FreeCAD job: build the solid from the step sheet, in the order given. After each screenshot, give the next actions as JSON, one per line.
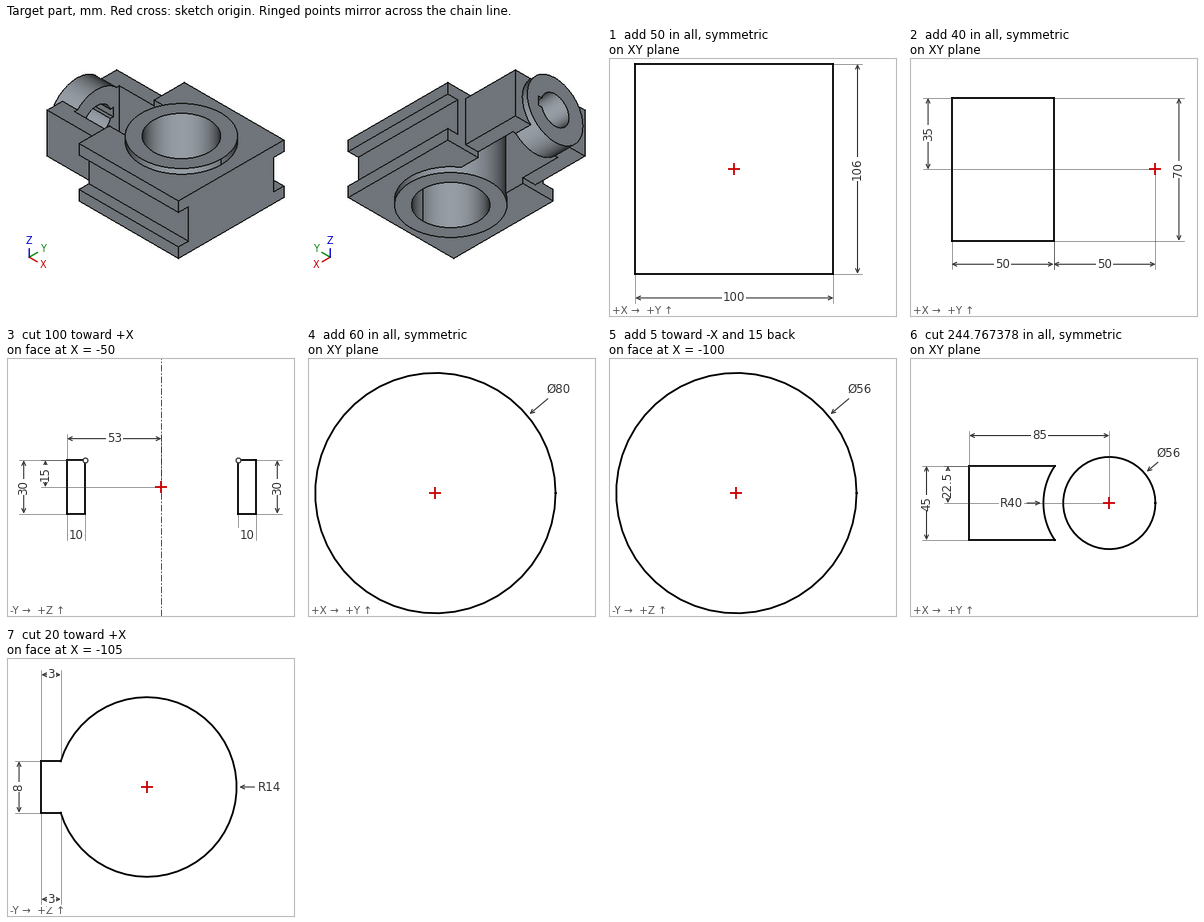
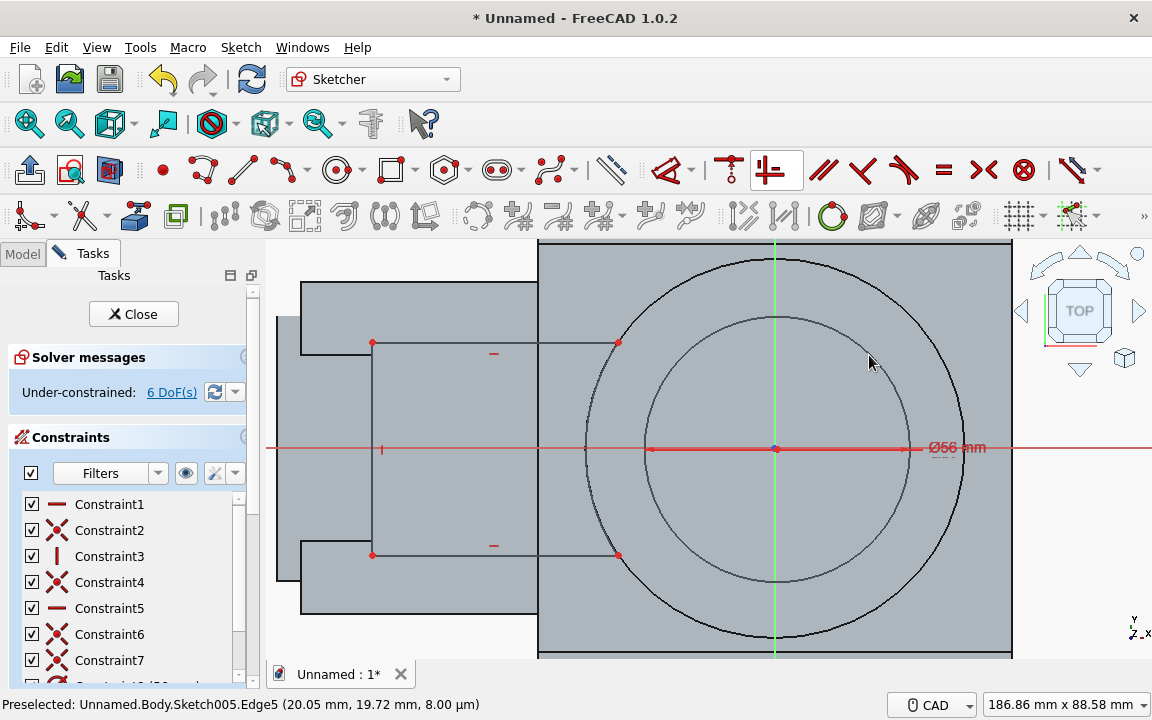
{"action": "left_click_drag", "start_coordinate": [765, 438], "coordinate": [787, 460]}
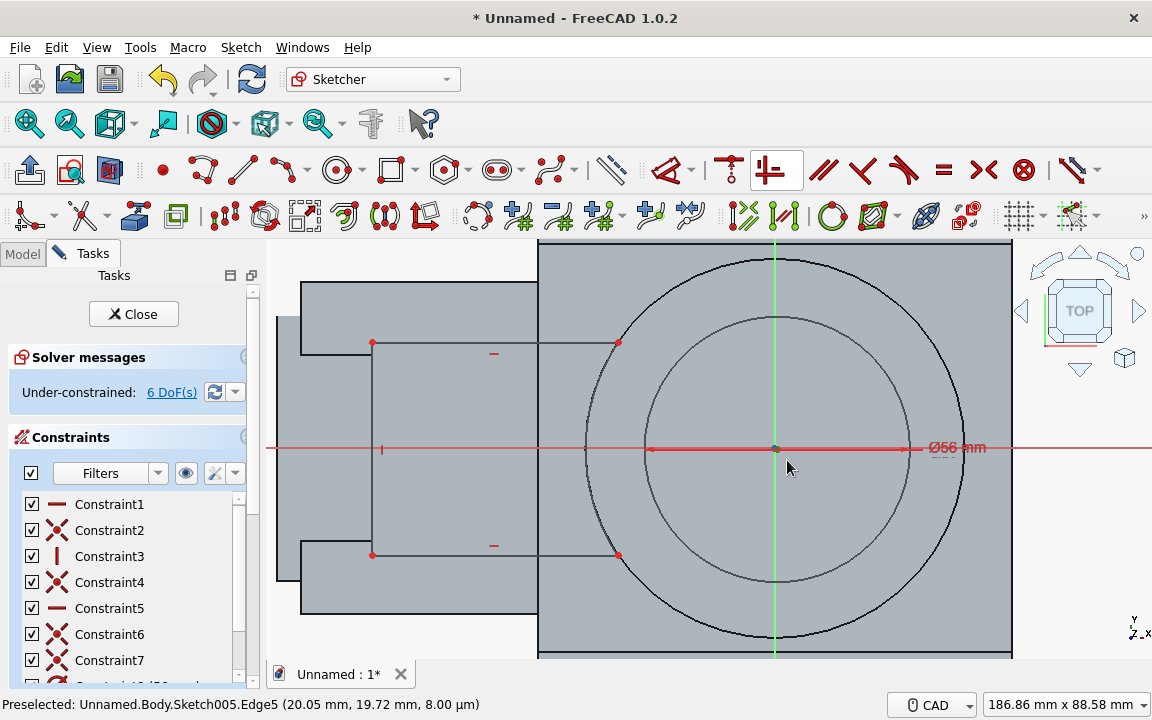
{"action": "left_click", "coordinate": [730, 170]}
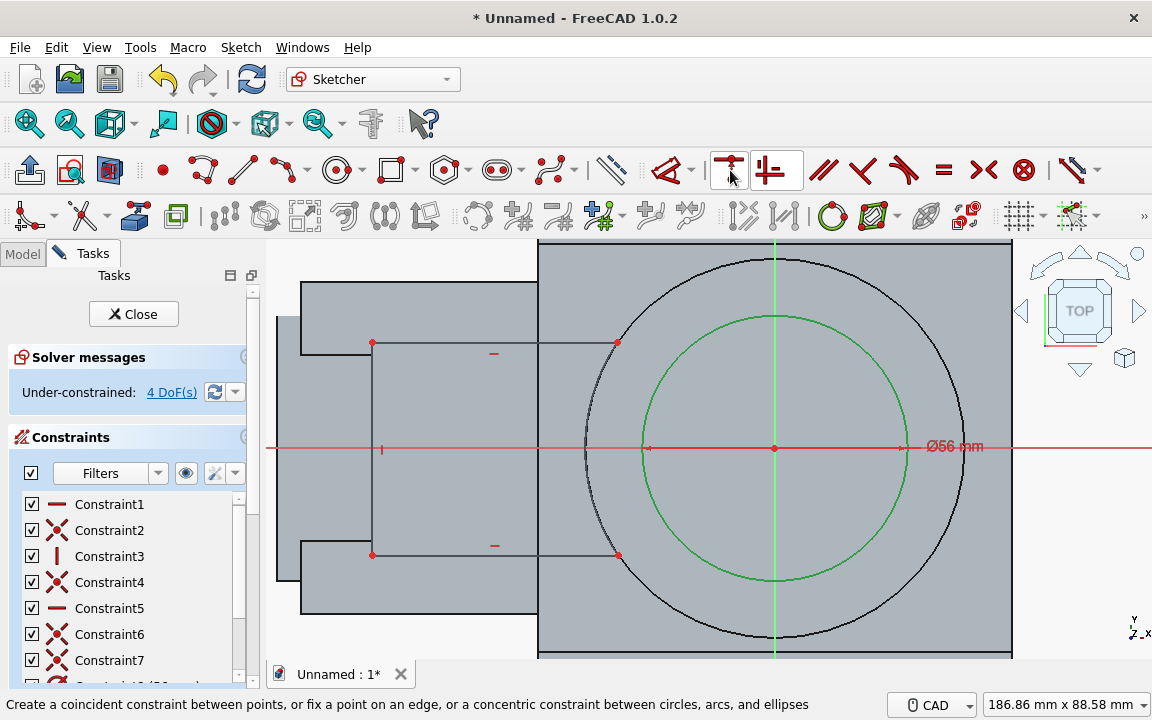
{"action": "left_click", "coordinate": [666, 170]}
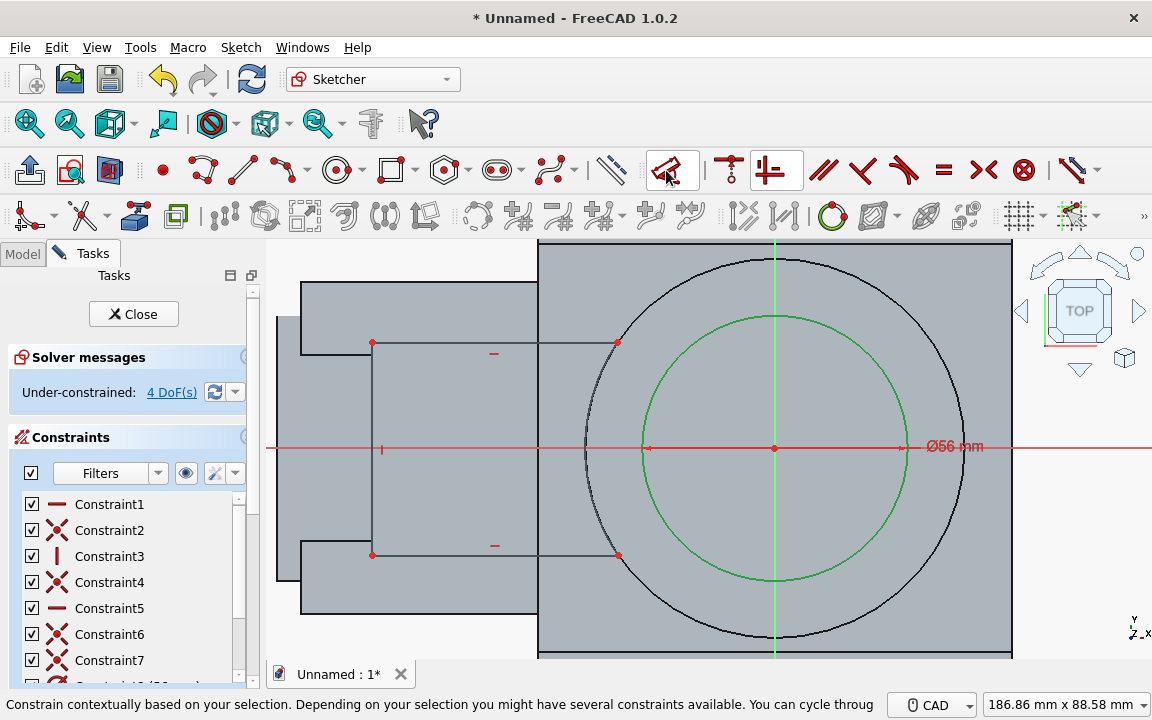
{"action": "left_click", "coordinate": [590, 405]}
{"action": "left_click", "coordinate": [559, 398]}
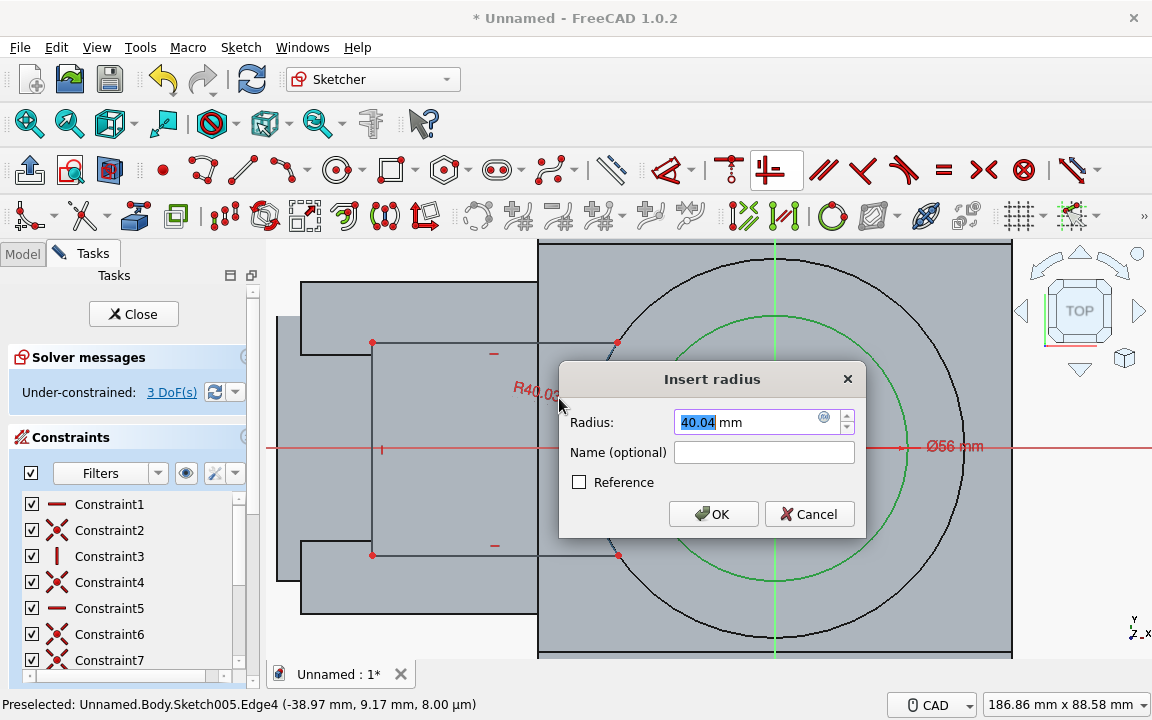
{"action": "type", "text": "40"}
{"action": "key", "text": "Return"}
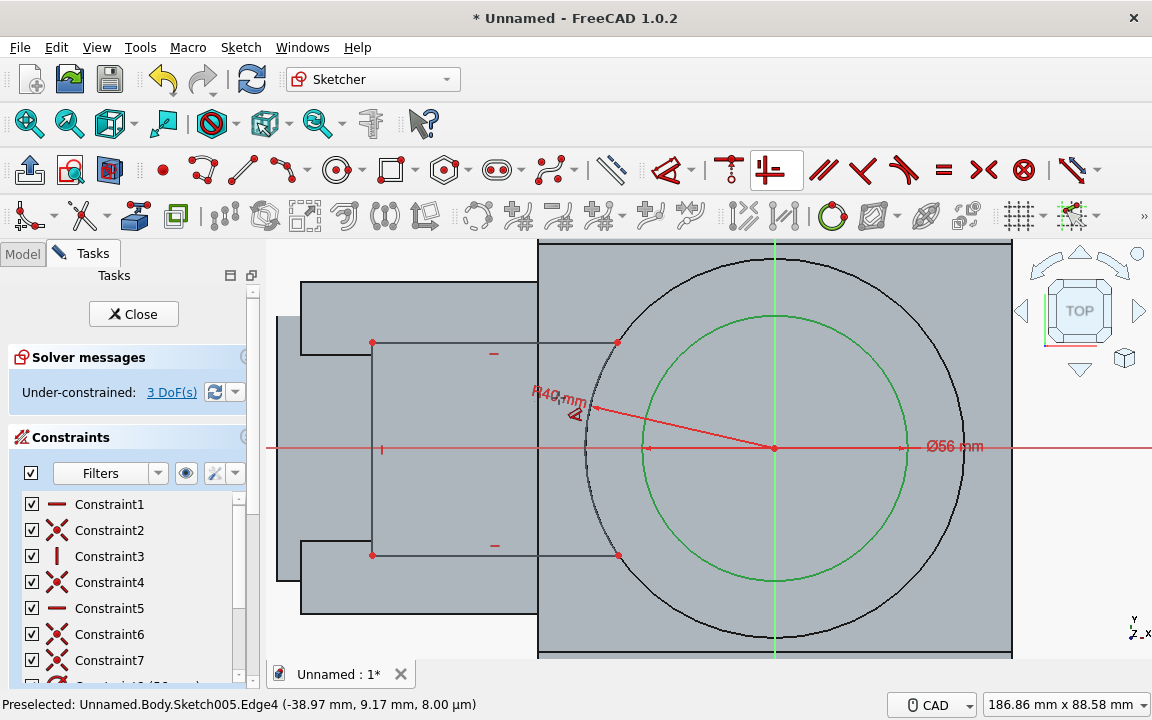
{"action": "left_click", "coordinate": [372, 407]}
{"action": "left_click", "coordinate": [338, 401]}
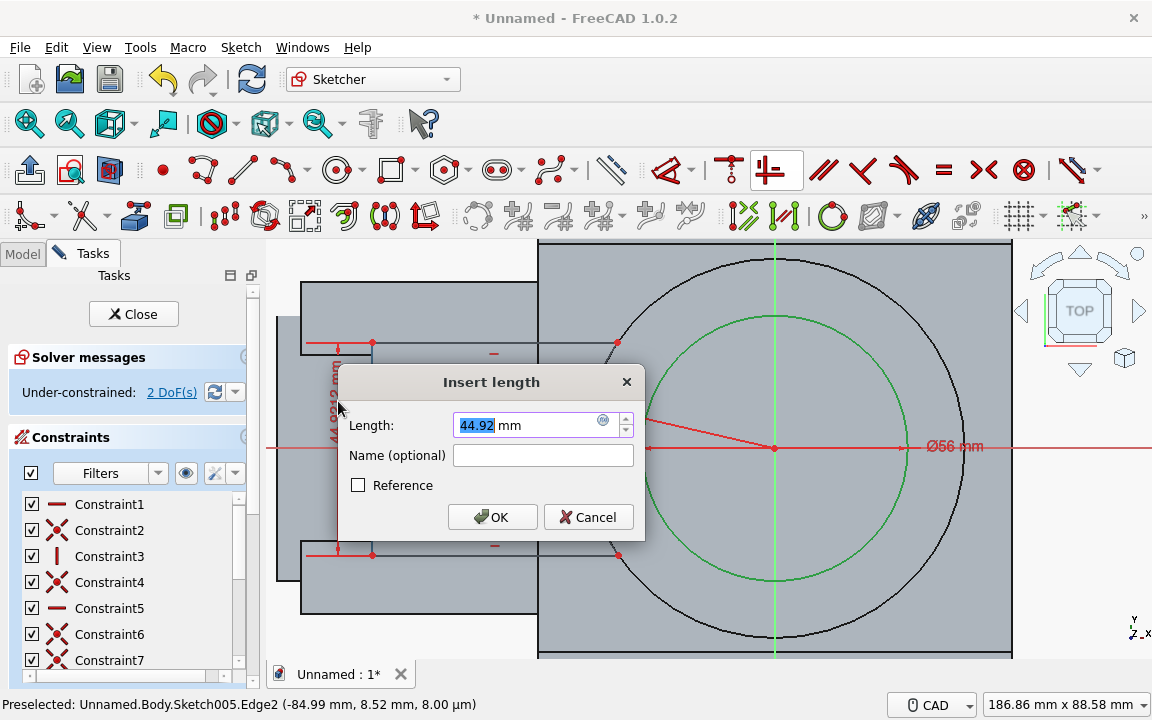
{"action": "type", "text": "45"}
{"action": "key", "text": "Return"}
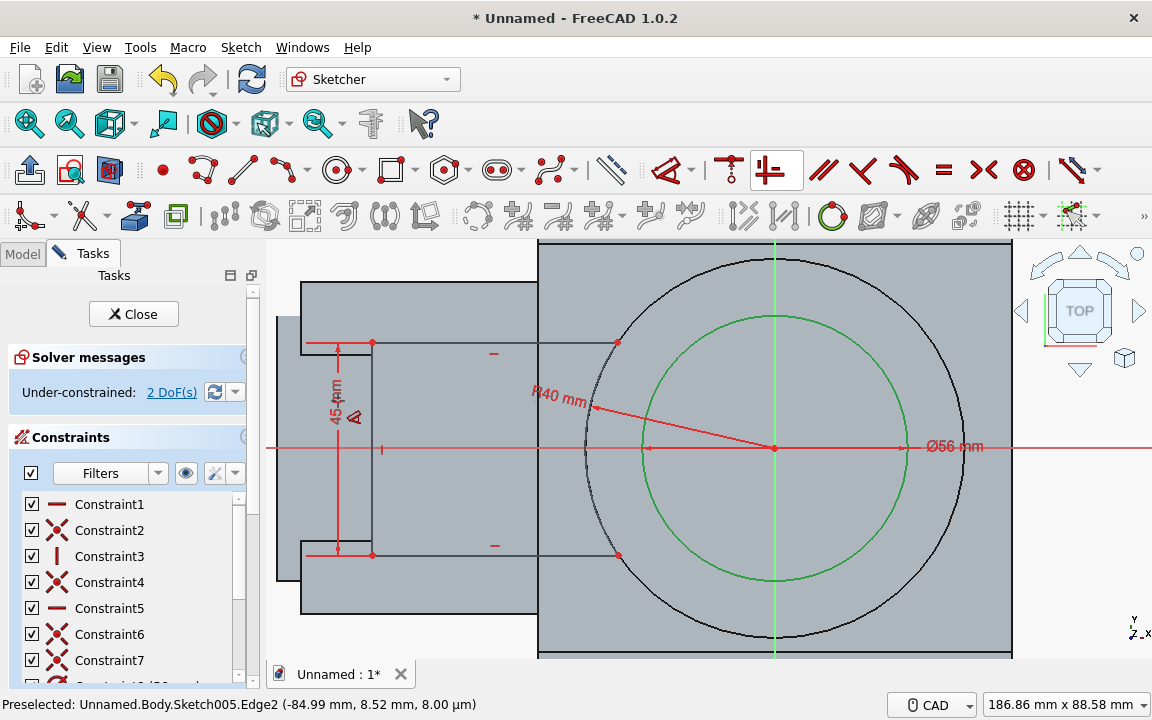
{"action": "left_click", "coordinate": [372, 343]}
{"action": "left_click", "coordinate": [573, 309]}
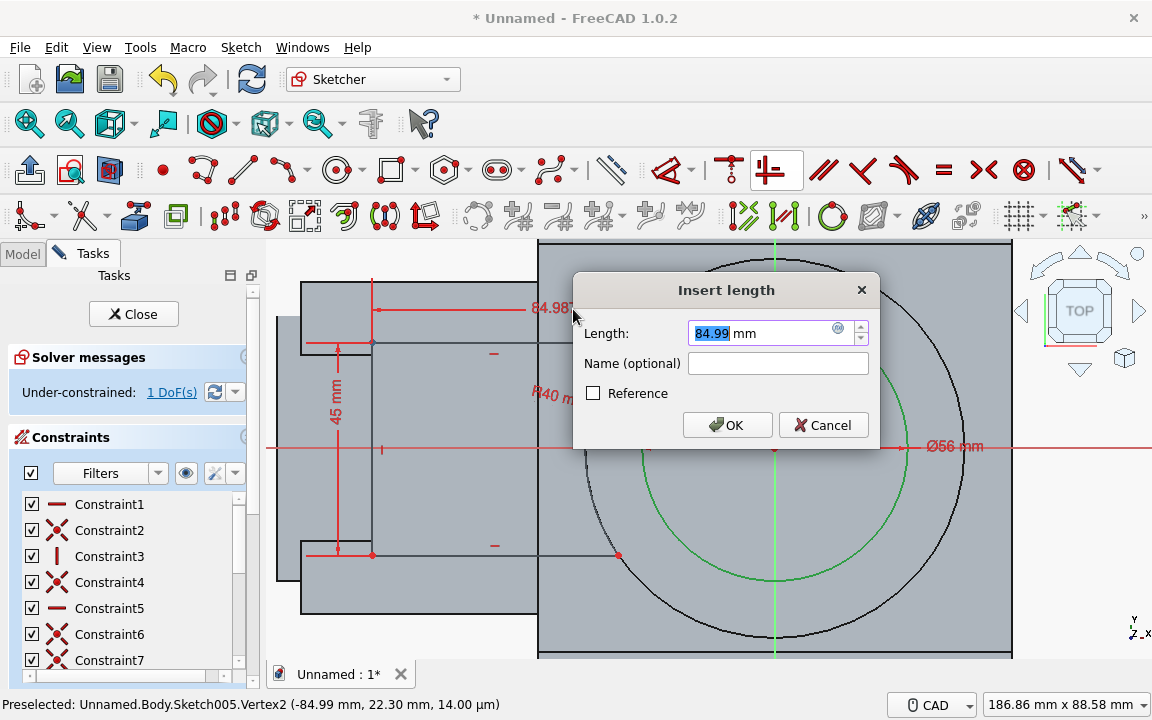
{"action": "type", "text": "85"}
{"action": "key", "text": "Return"}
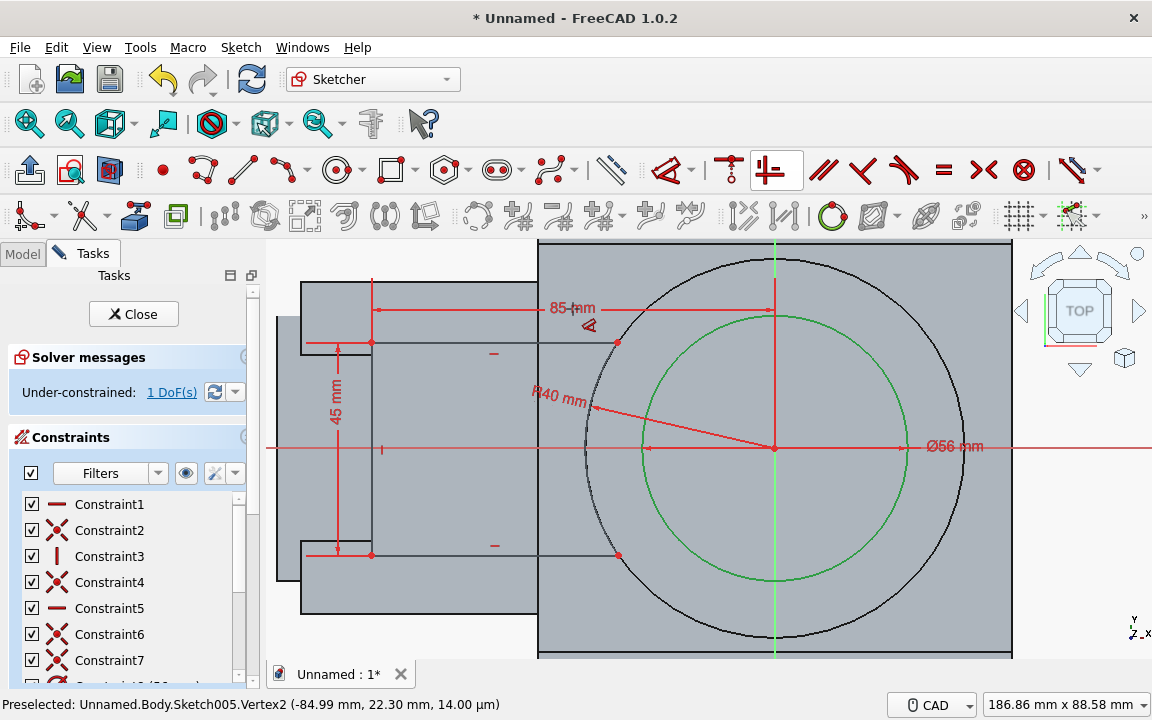
{"action": "left_click", "coordinate": [618, 343]}
{"action": "left_click", "coordinate": [809, 396]}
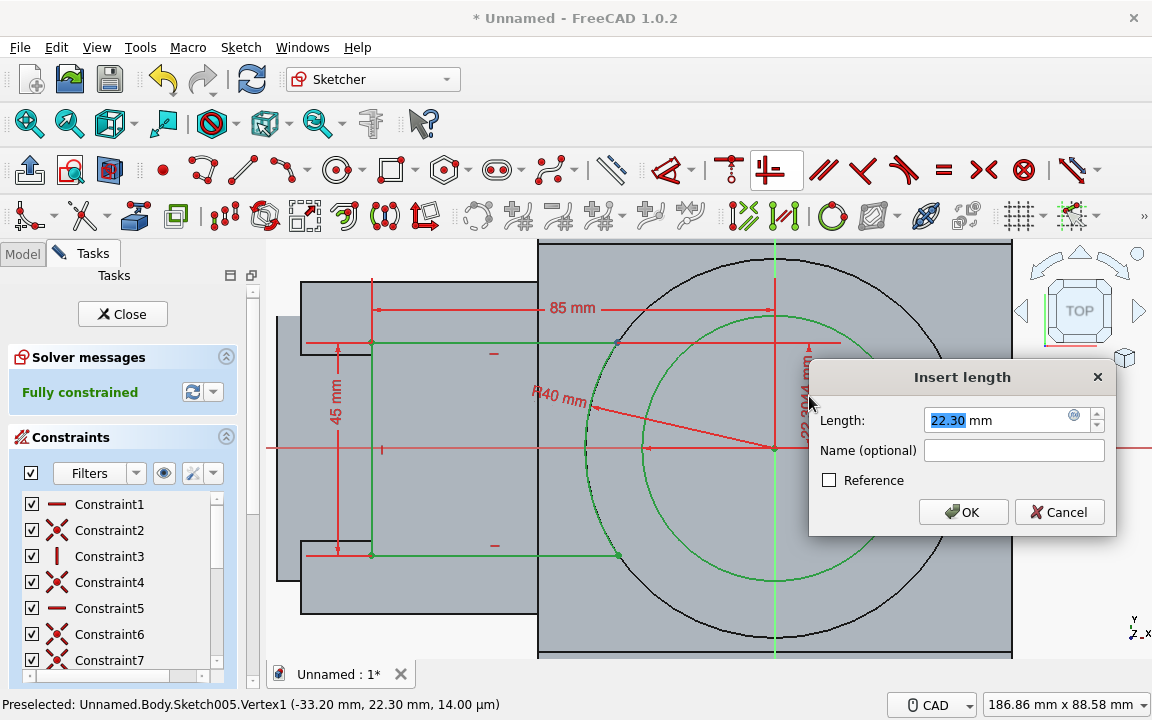
{"action": "type", "text": "22.5"}
{"action": "key", "text": "Return"}
{"action": "key", "text": "Escape"}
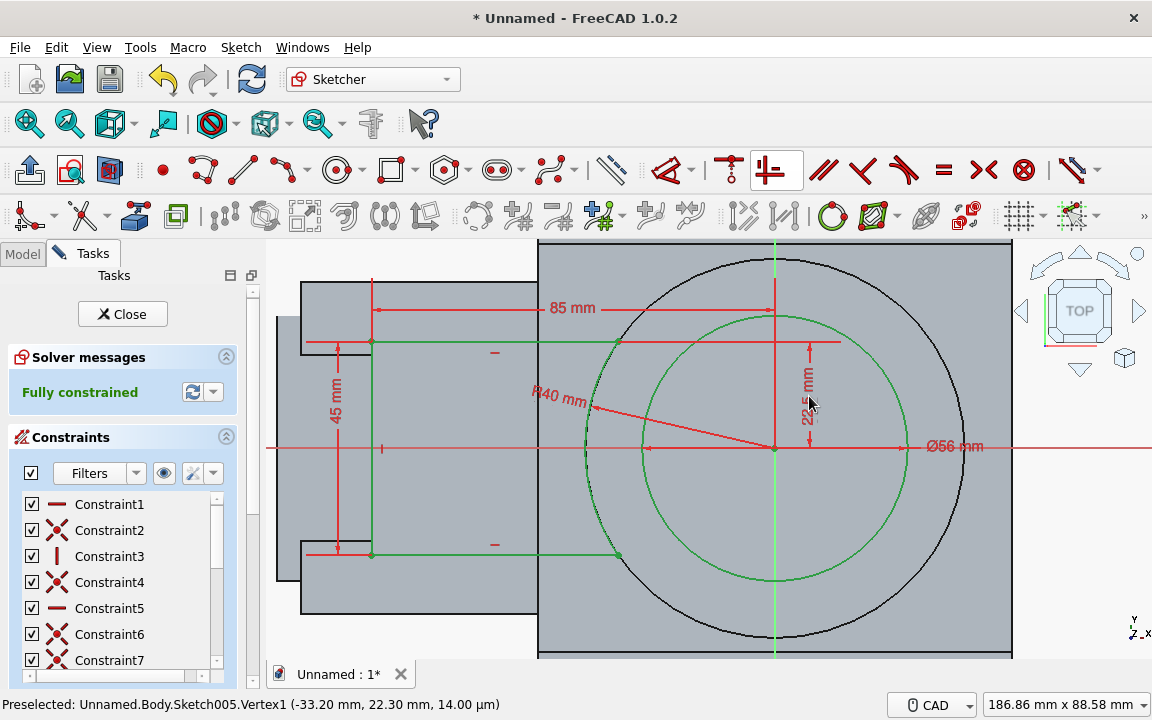
{"action": "left_click", "coordinate": [123, 314]}